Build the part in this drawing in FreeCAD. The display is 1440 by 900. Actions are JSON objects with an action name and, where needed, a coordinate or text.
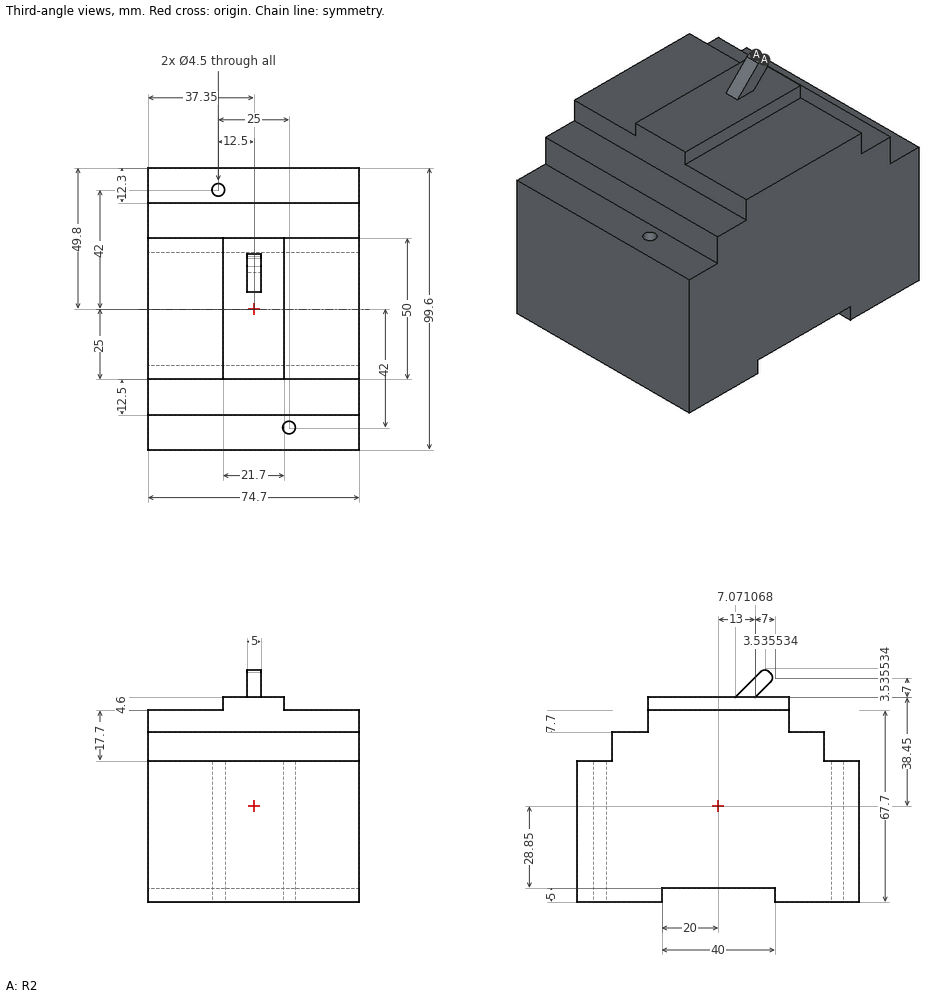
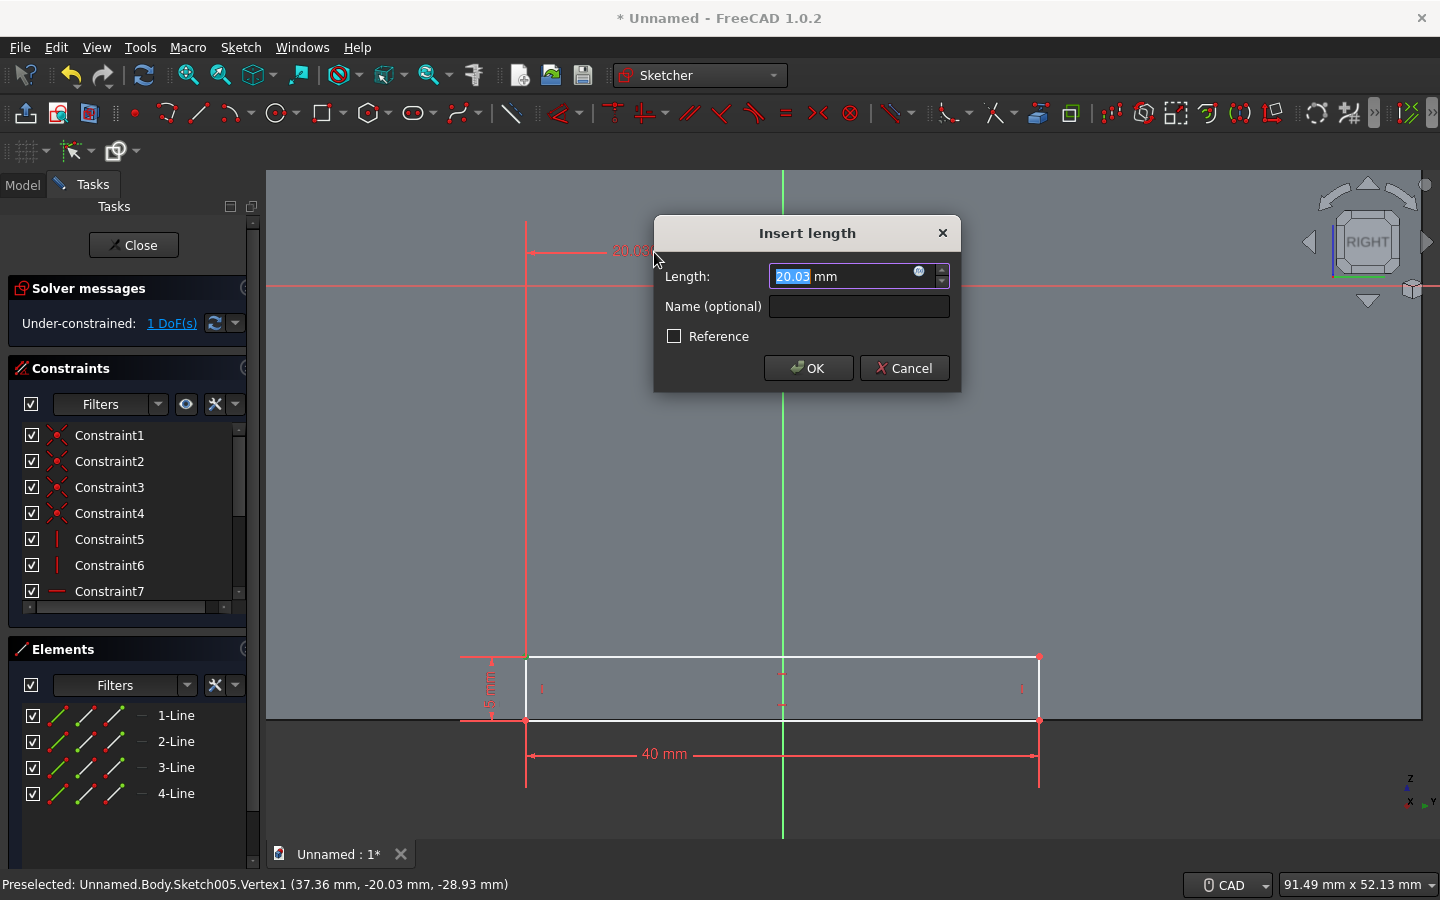
{"action": "type", "text": "20"}
{"action": "key", "text": "Return"}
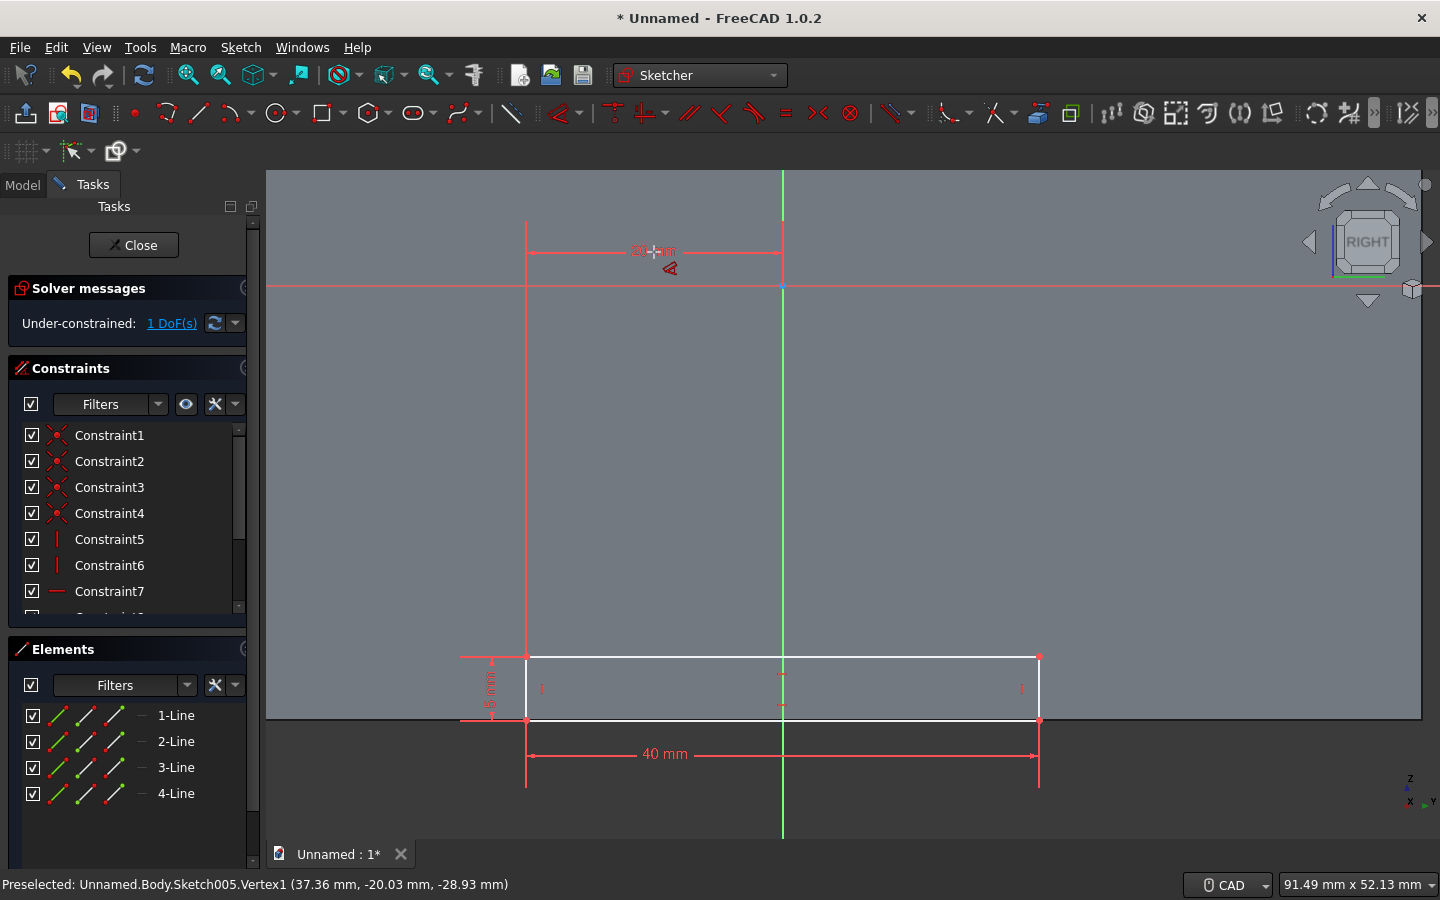
{"action": "left_click", "coordinate": [526, 657]}
{"action": "left_click", "coordinate": [492, 471]}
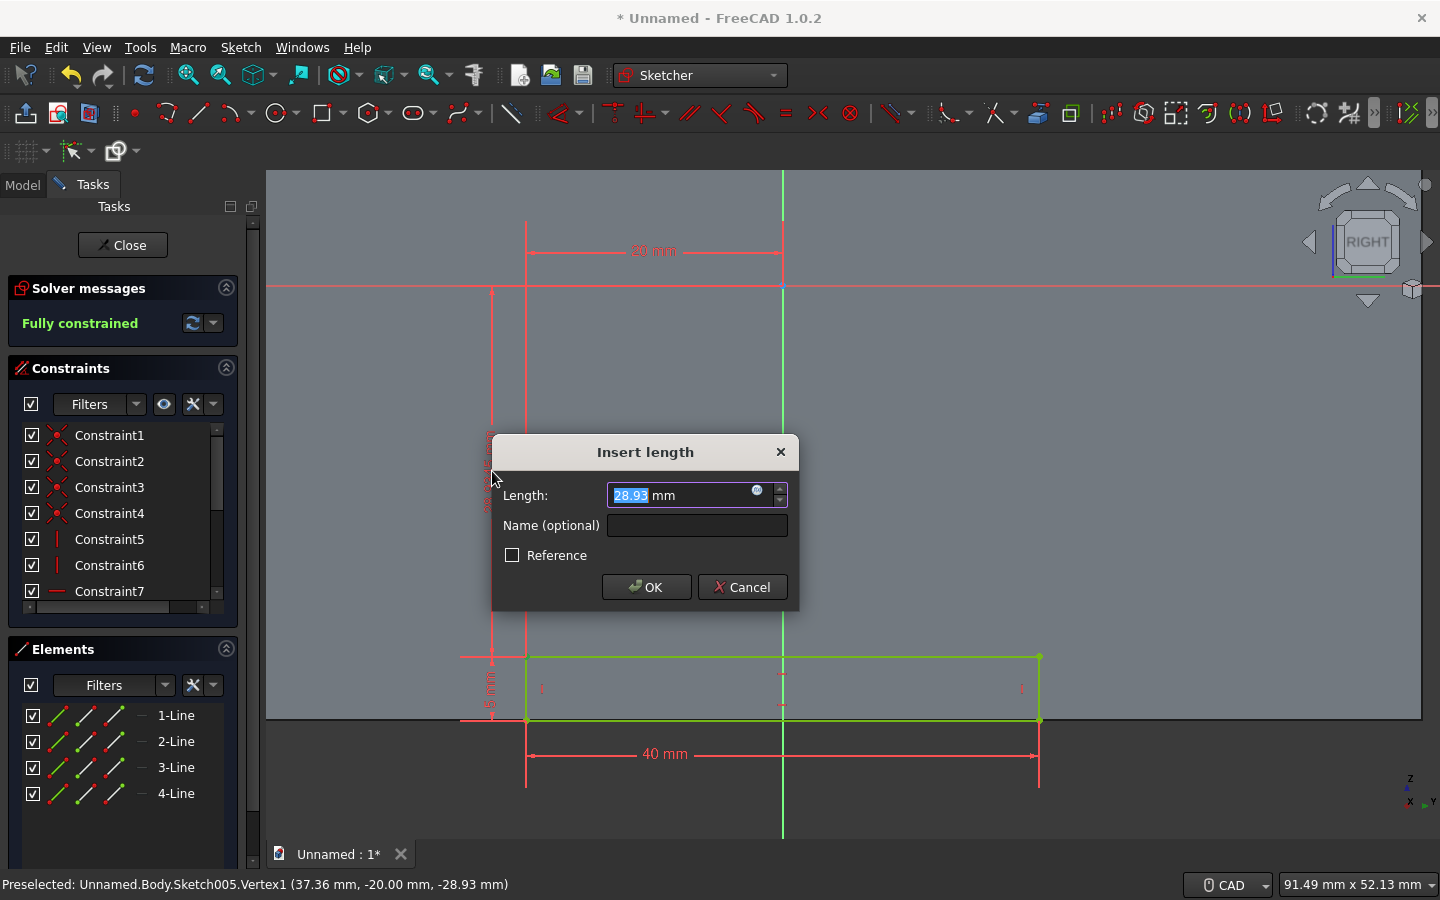
{"action": "type", "text": "28.85"}
{"action": "key", "text": "Return"}
{"action": "key", "text": "Escape"}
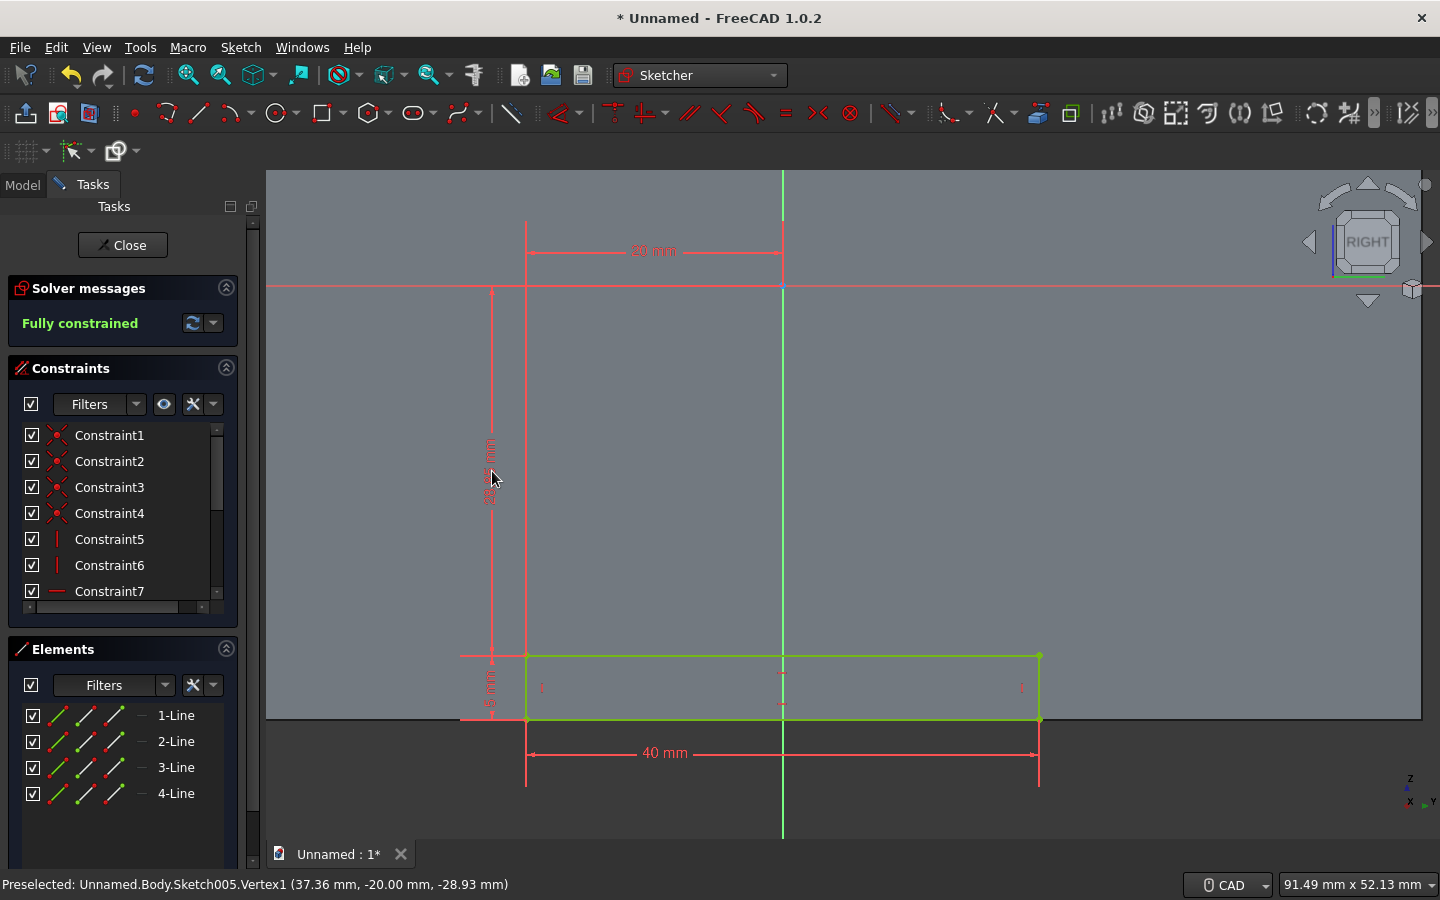
{"action": "left_click", "coordinate": [123, 245]}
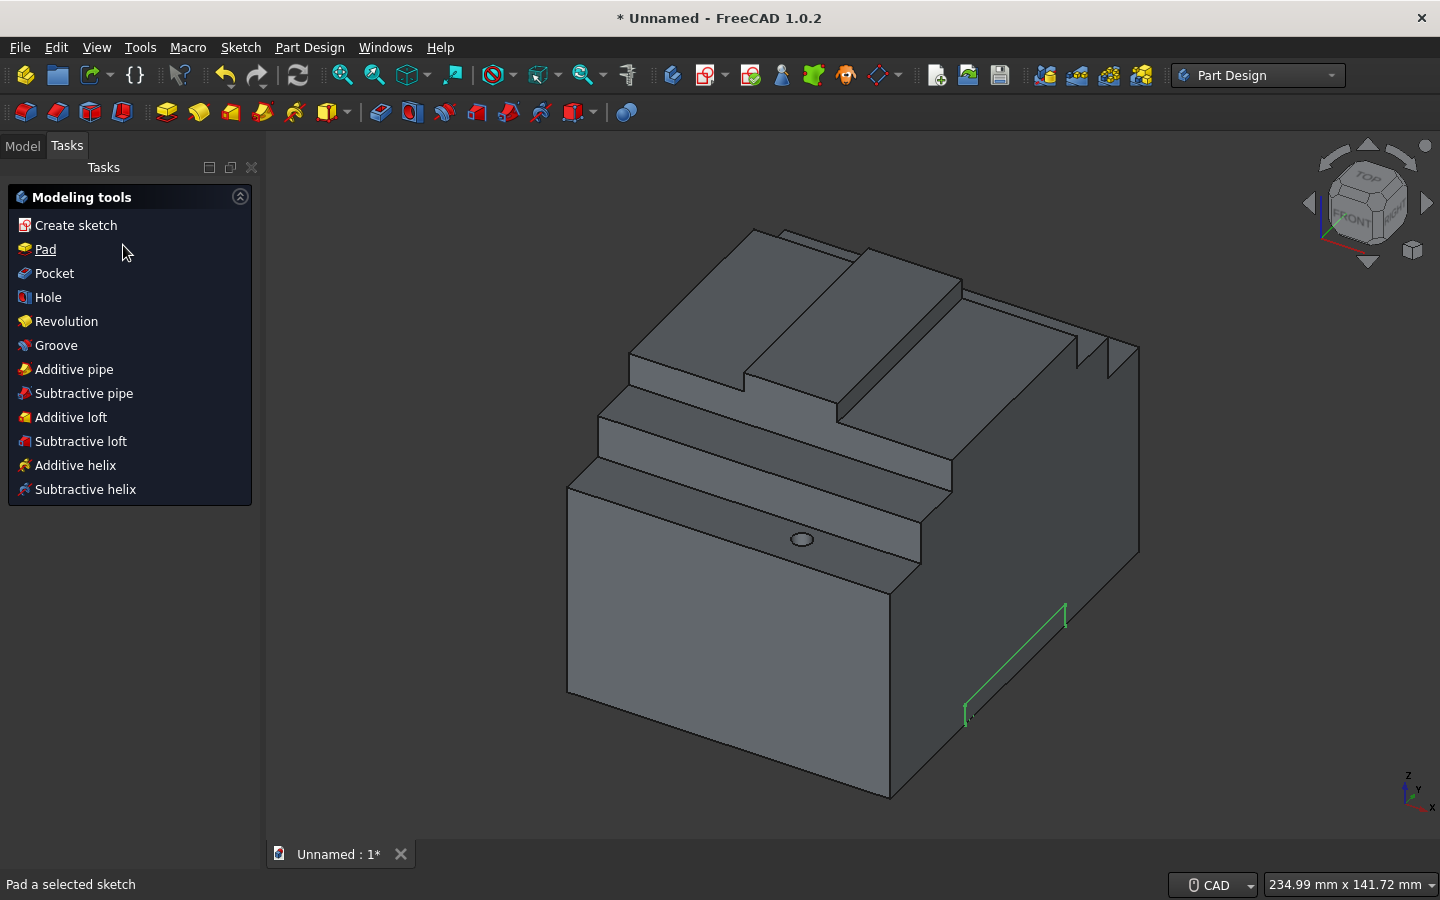
{"action": "left_click", "coordinate": [382, 112]}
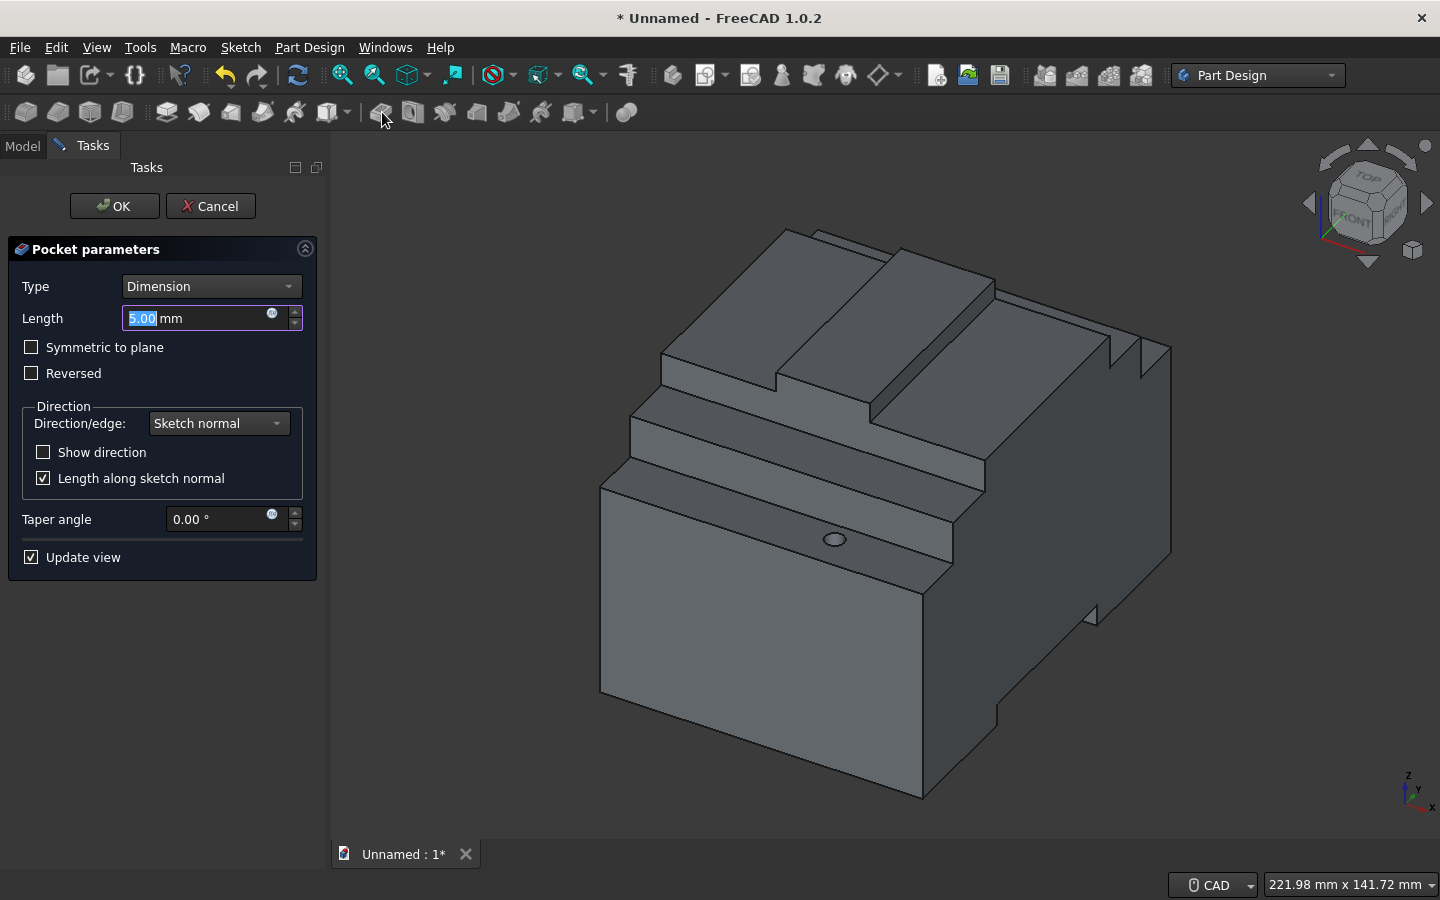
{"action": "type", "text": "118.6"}
{"action": "key", "text": "Tab"}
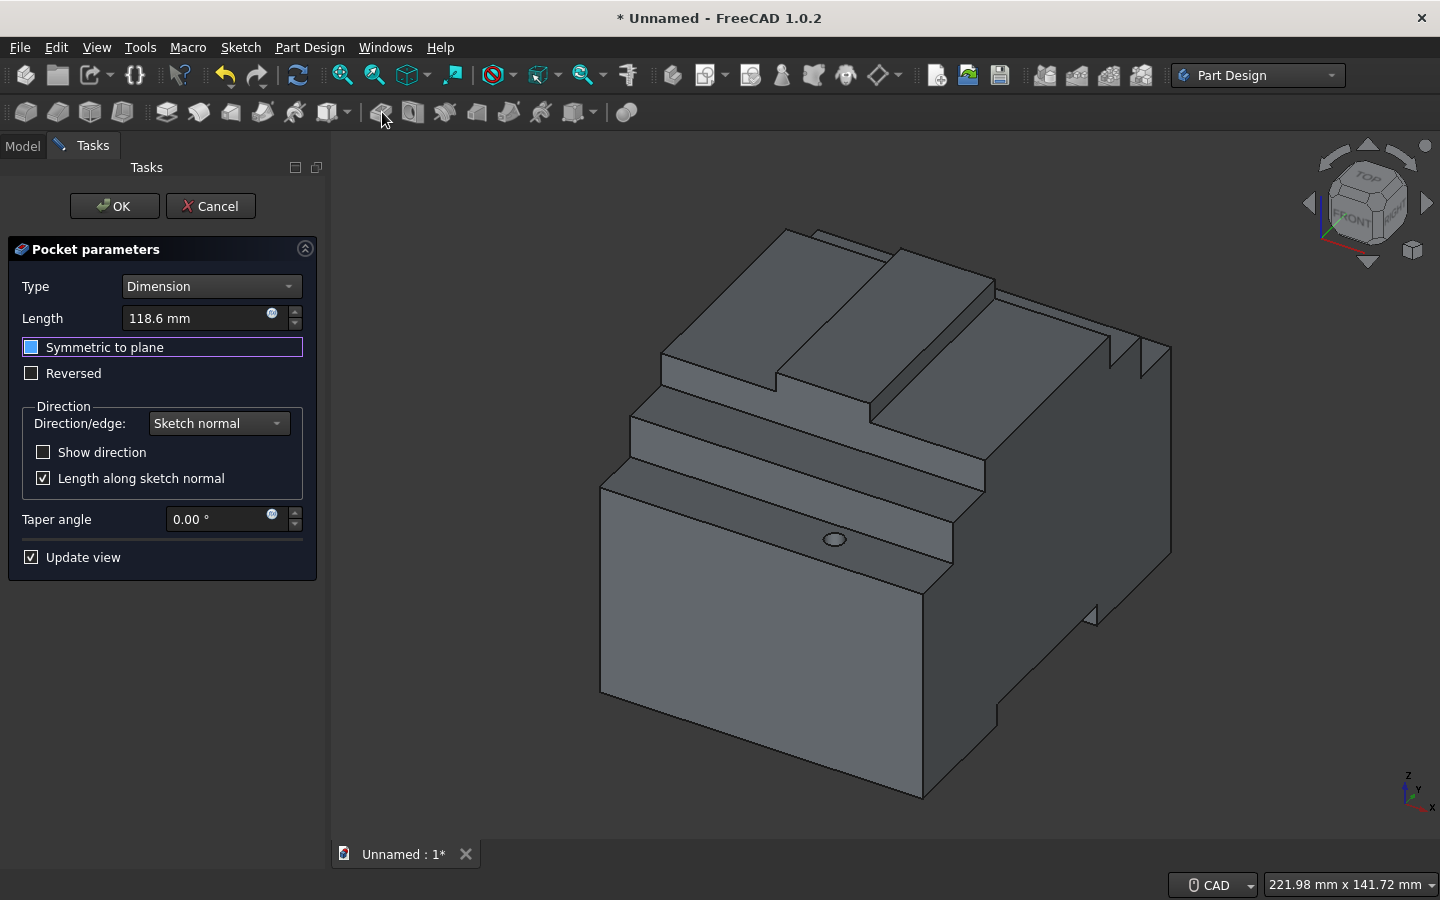
{"action": "left_click", "coordinate": [115, 206]}